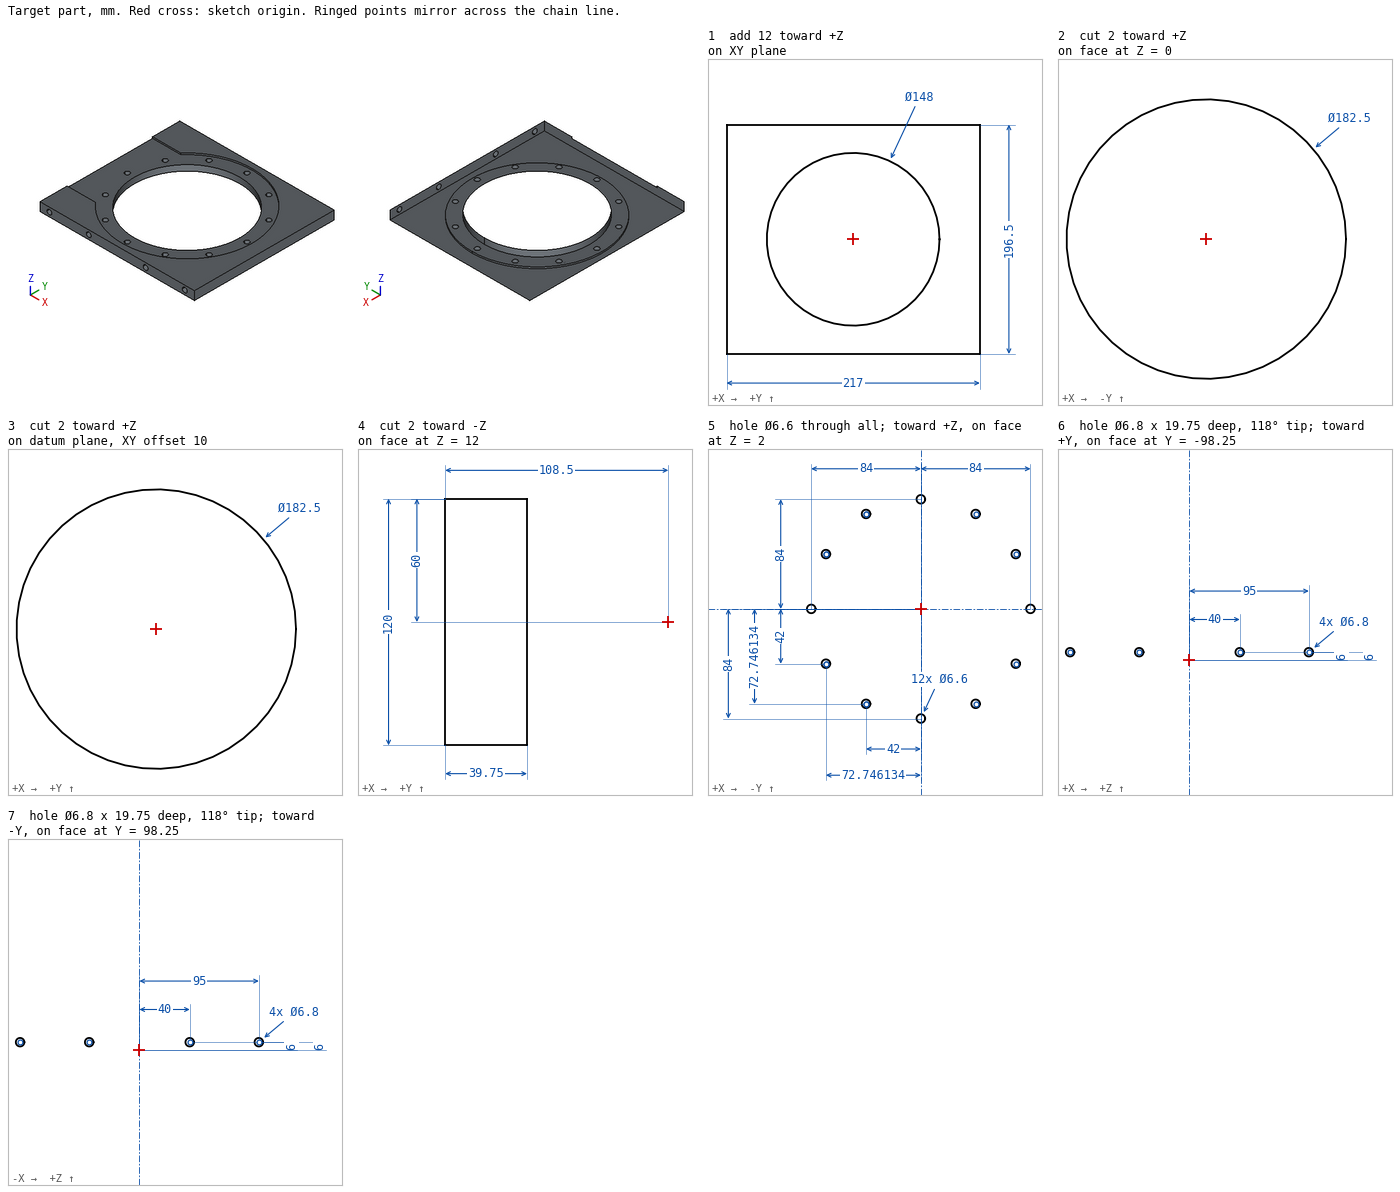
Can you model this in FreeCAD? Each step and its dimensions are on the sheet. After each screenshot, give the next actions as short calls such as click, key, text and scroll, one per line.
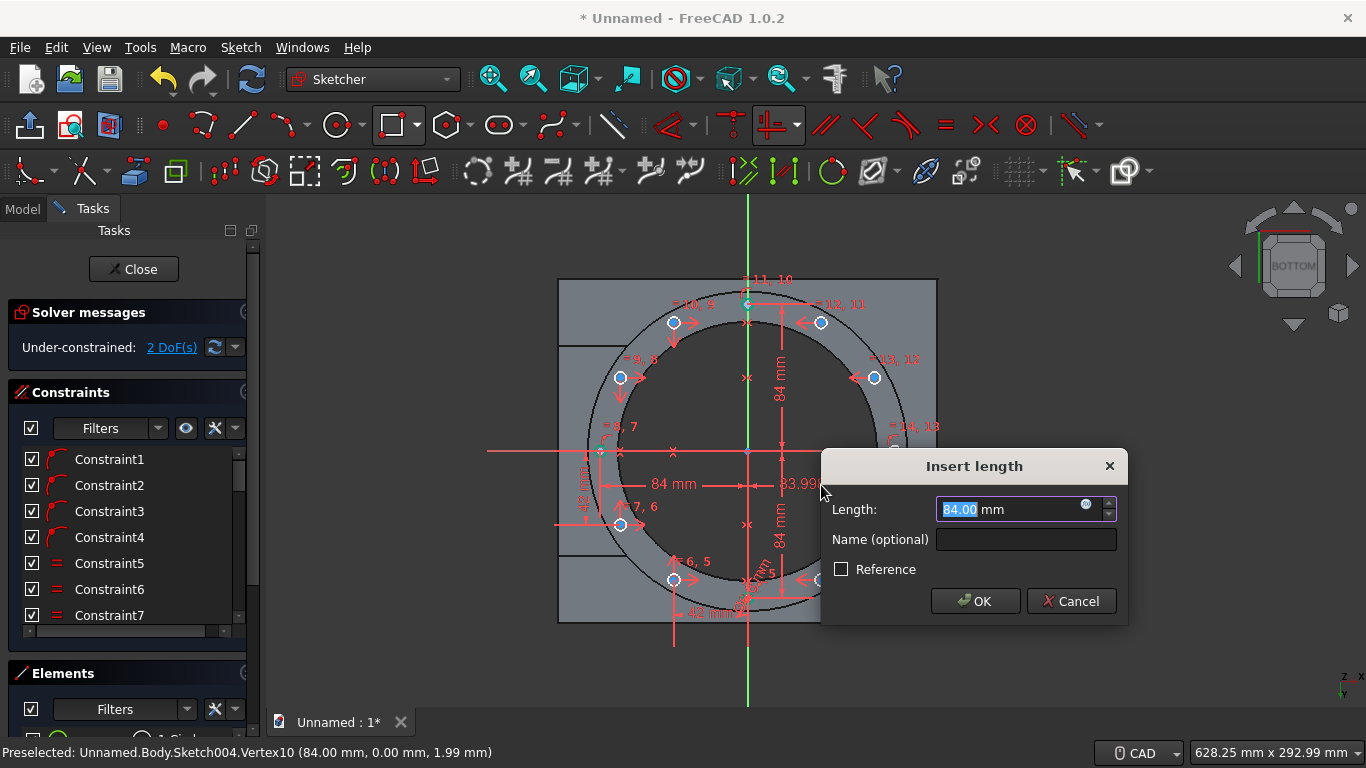
text(84)
key(Return)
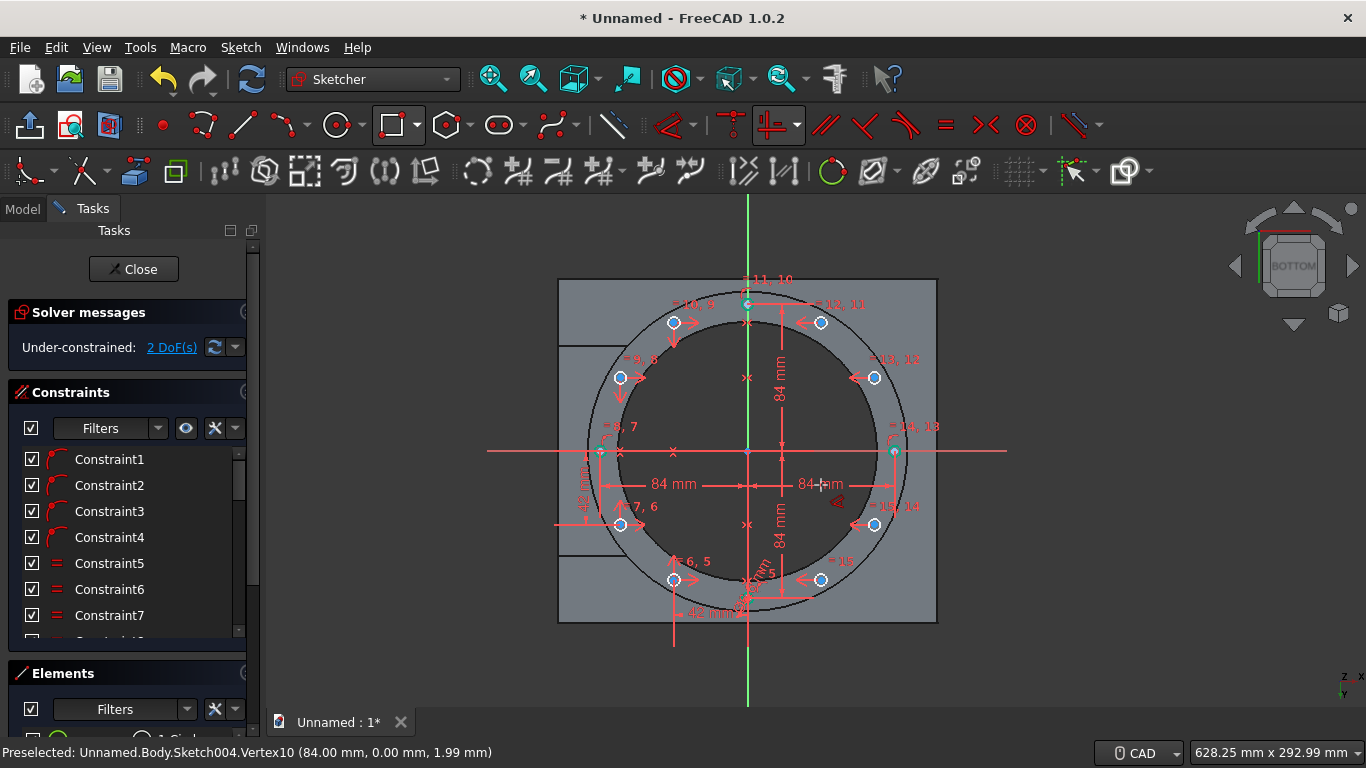
click(674, 580)
click(640, 516)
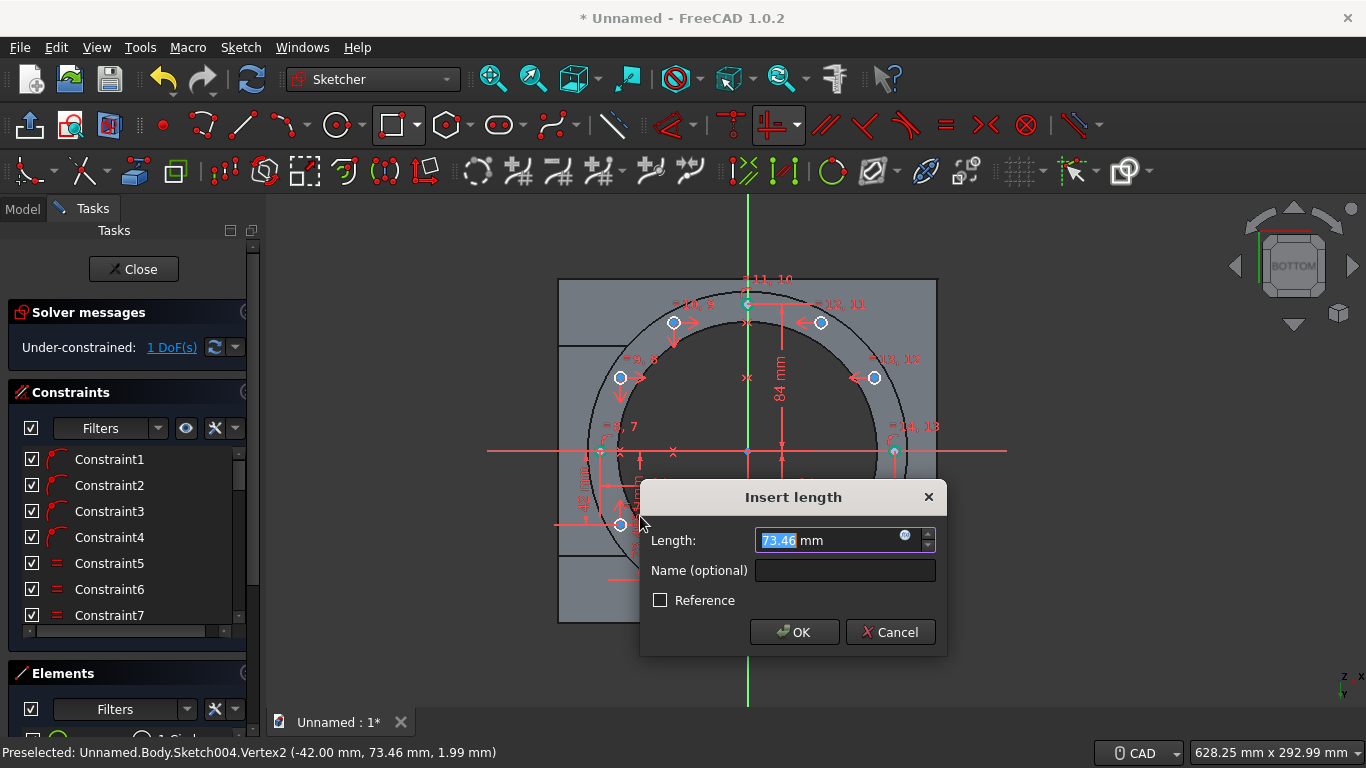
text(72.746134)
key(Return)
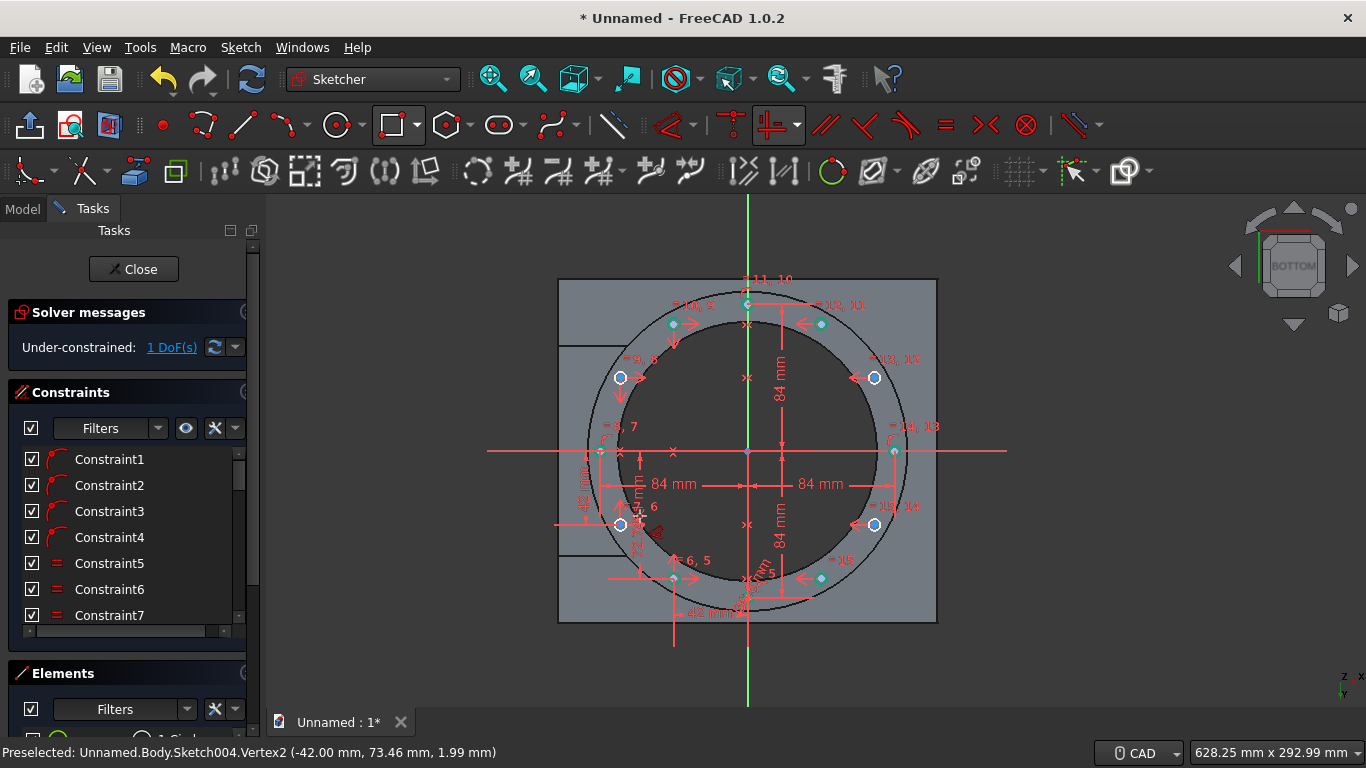
click(620, 525)
click(684, 559)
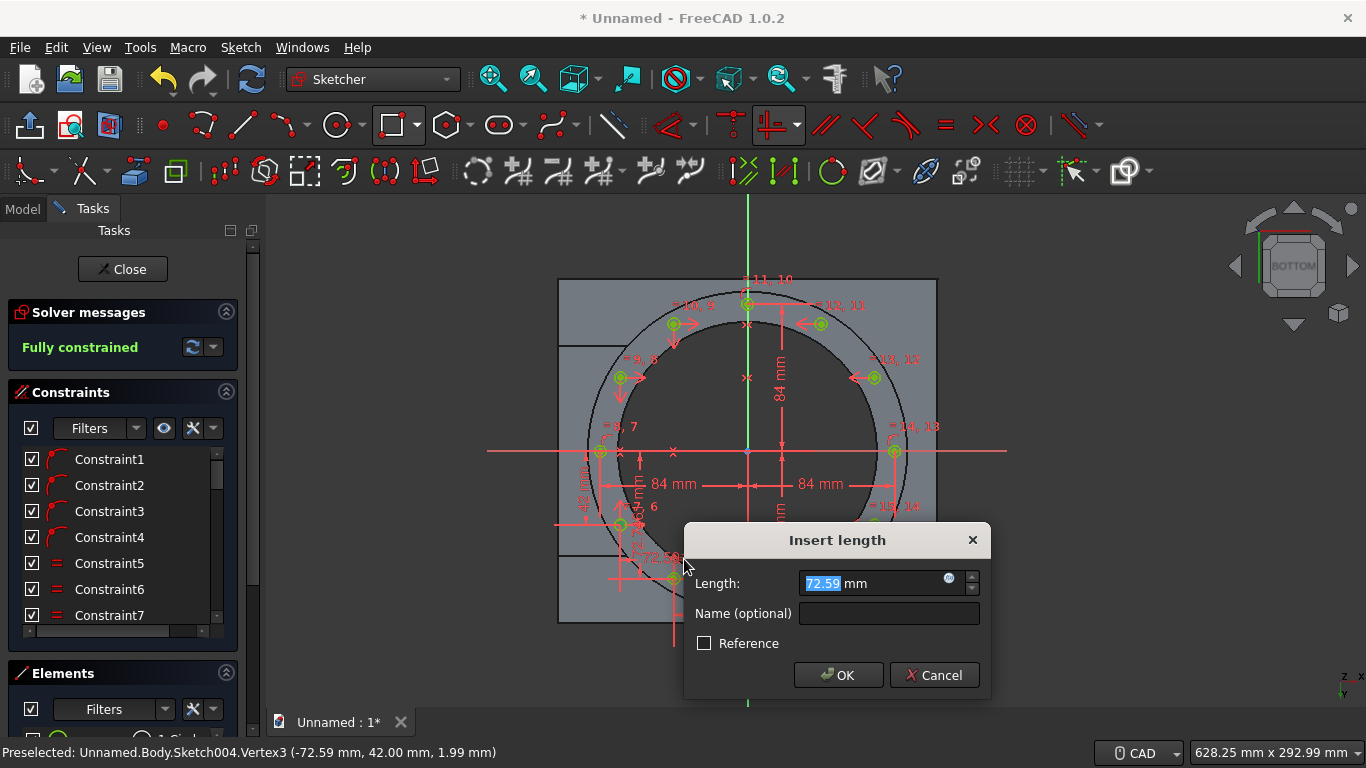
text(72.746134)
key(Return)
key(Escape)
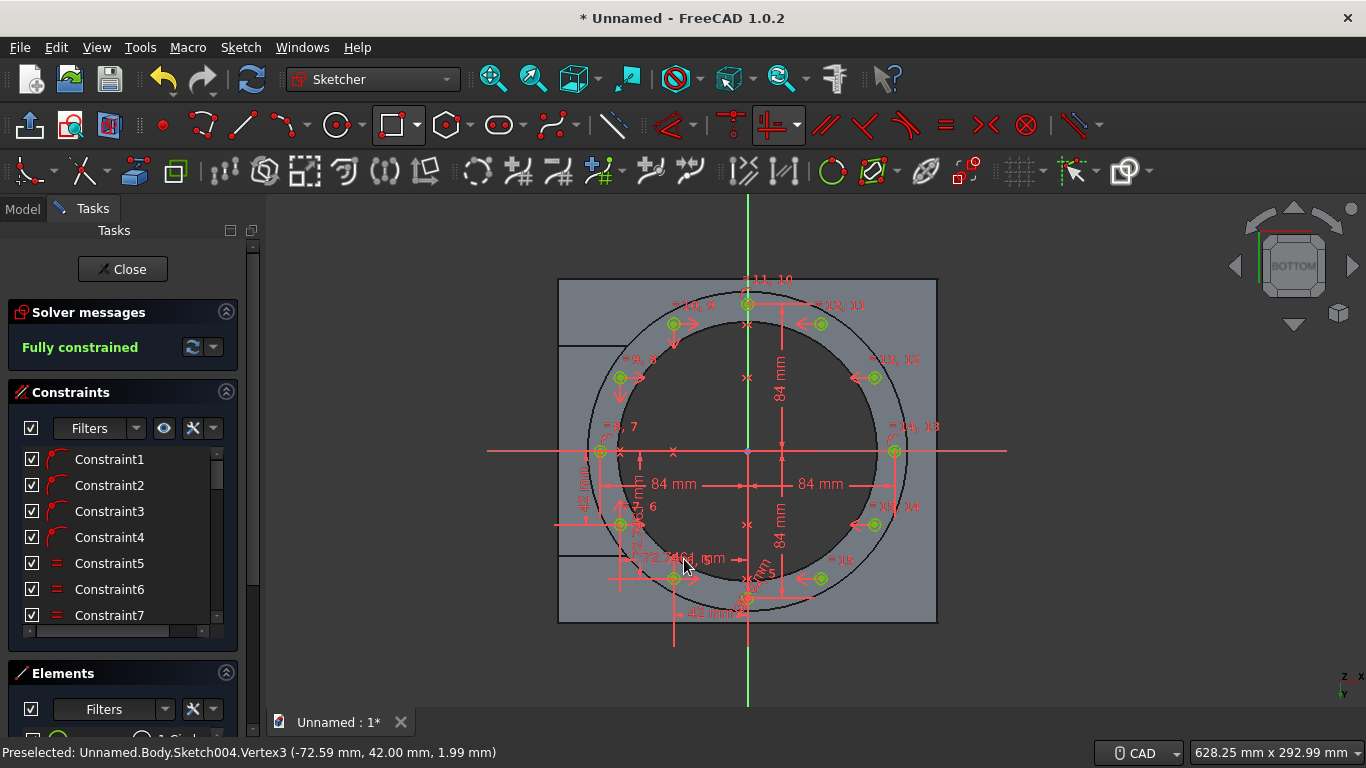
click(123, 269)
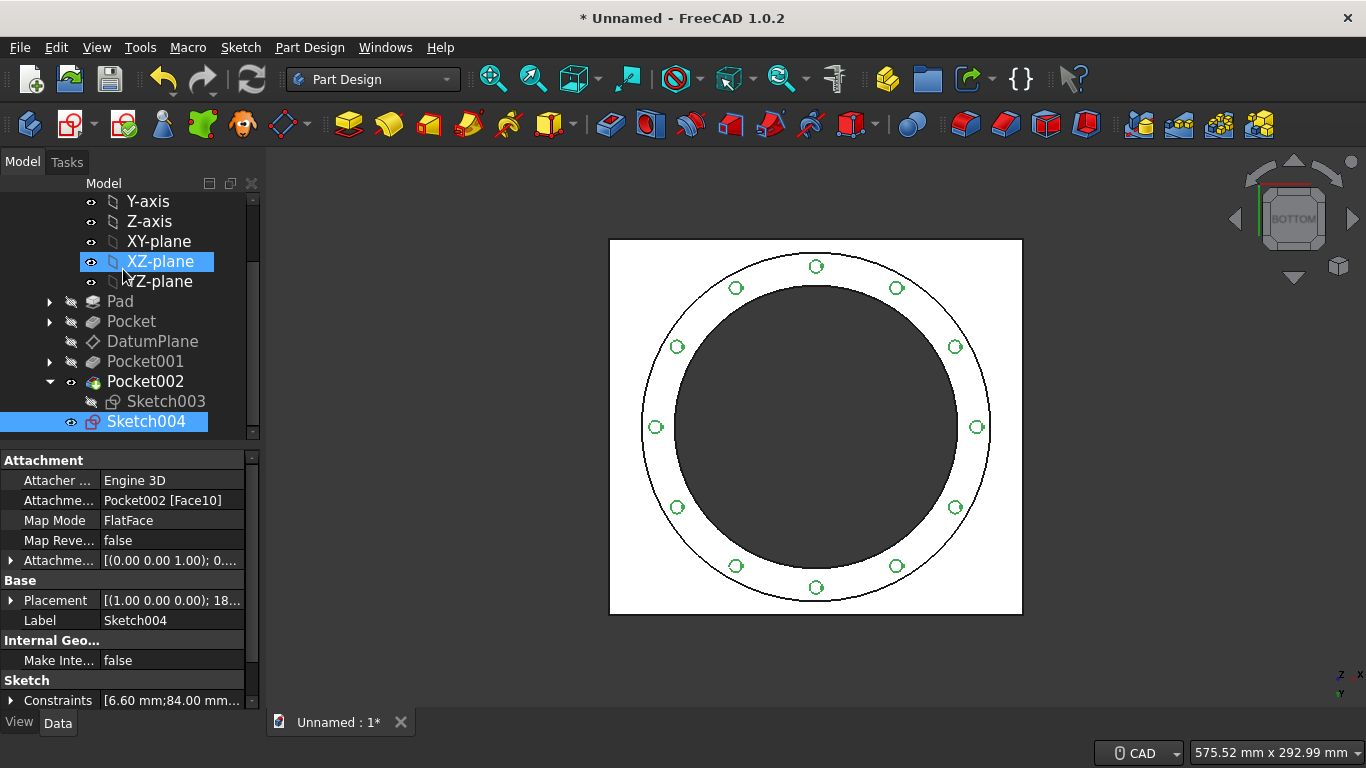
click(652, 124)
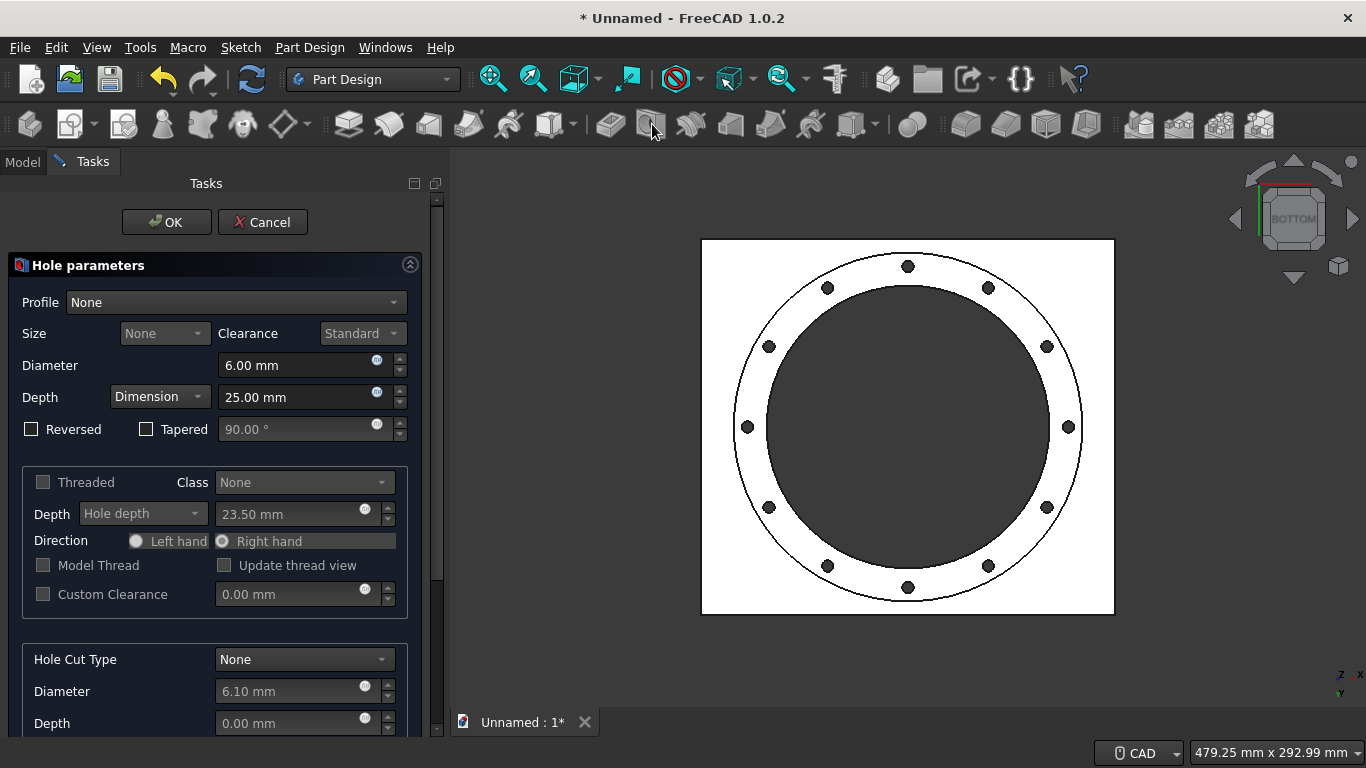
triple_click(305, 365)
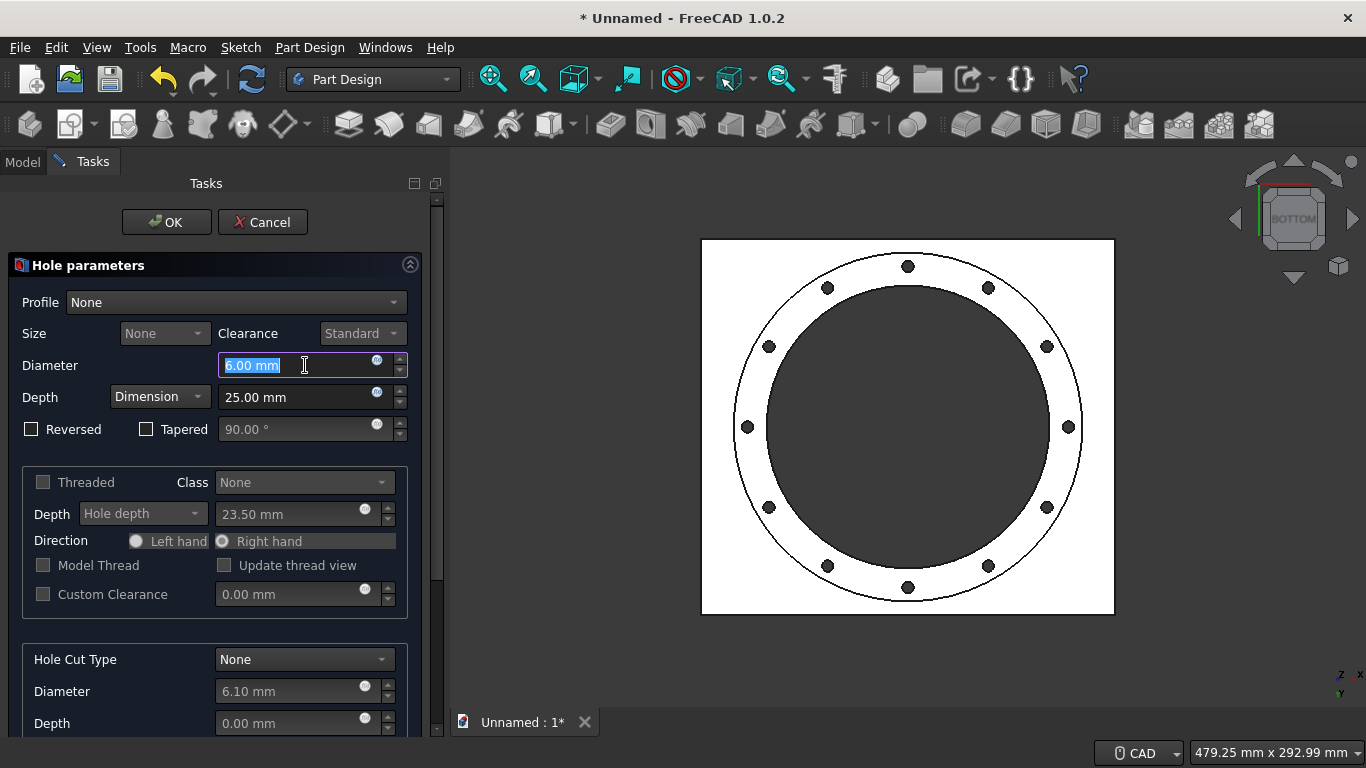
text(6.6)
key(Tab)